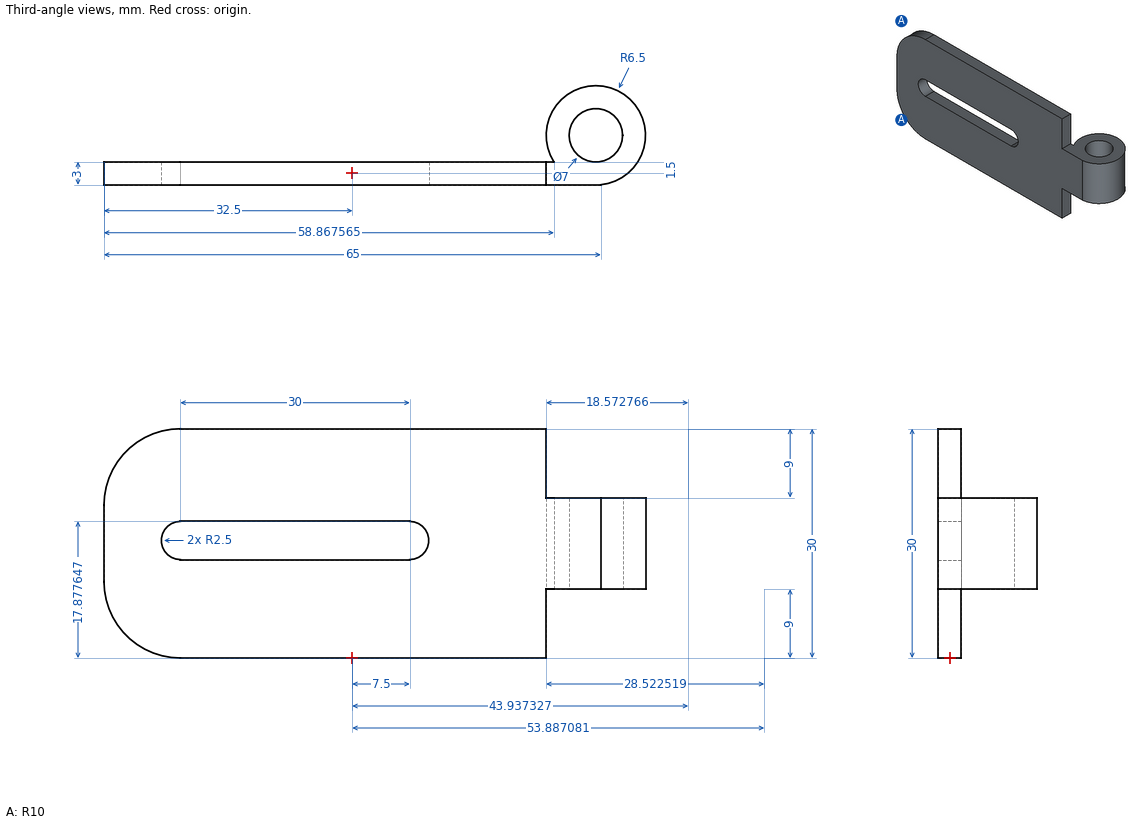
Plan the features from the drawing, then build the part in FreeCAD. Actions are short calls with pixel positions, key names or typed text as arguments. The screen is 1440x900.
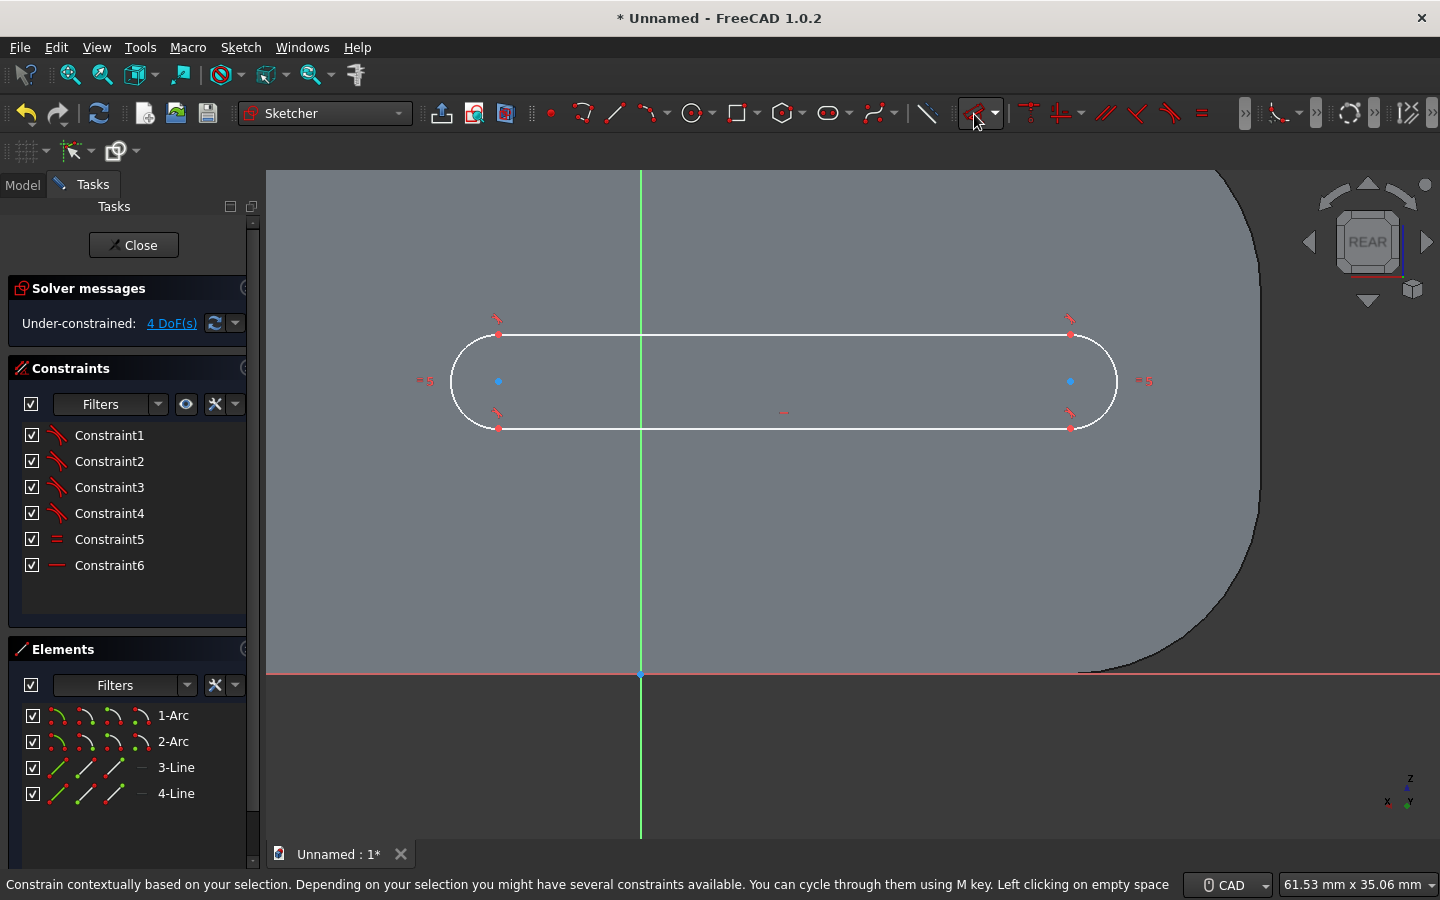
click(460, 354)
click(434, 335)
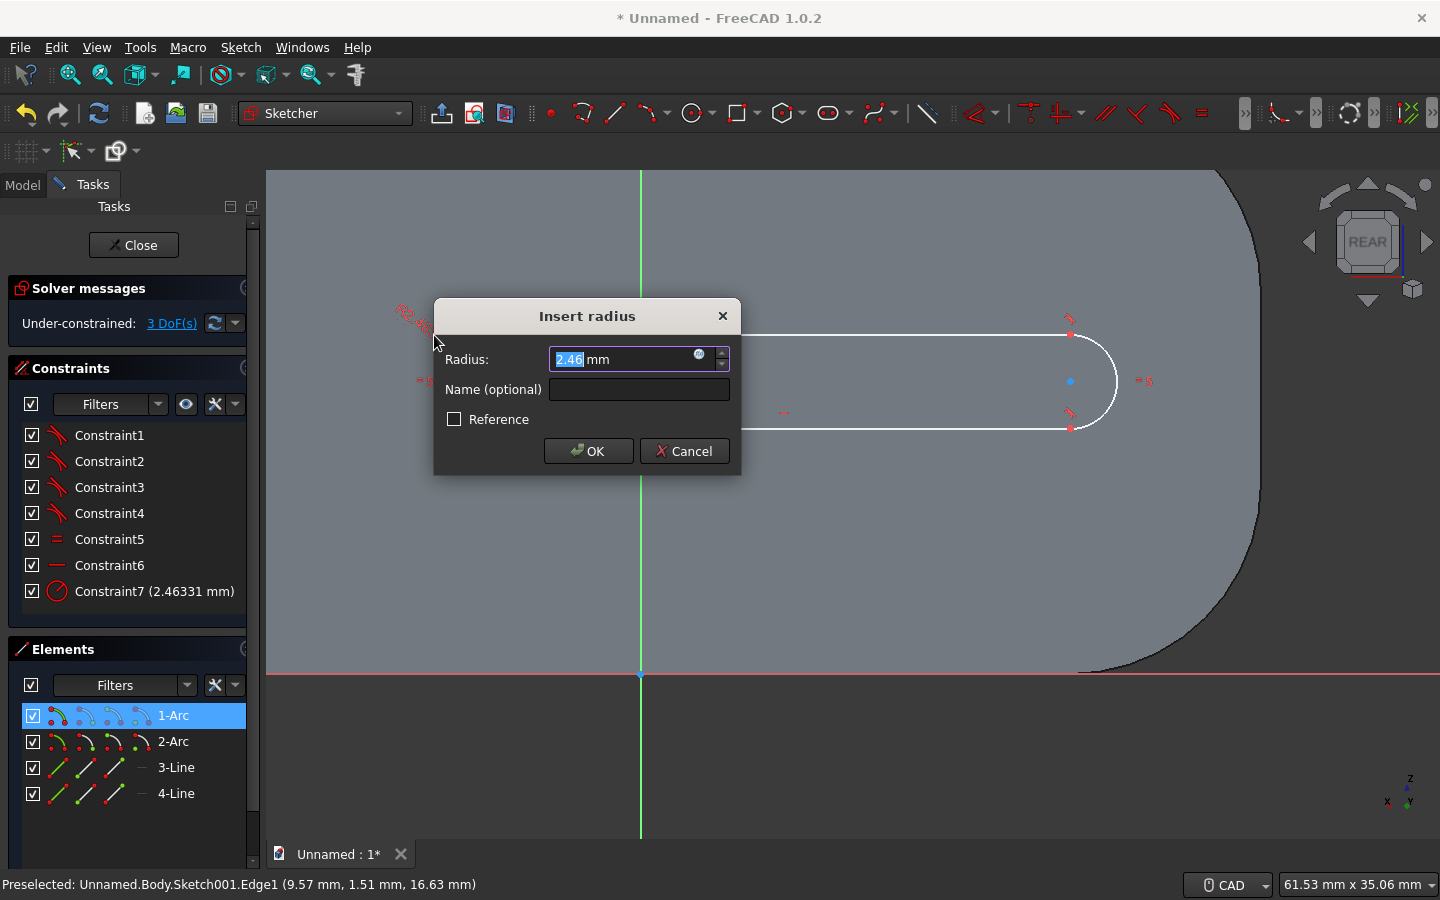
text(2.5)
key(Return)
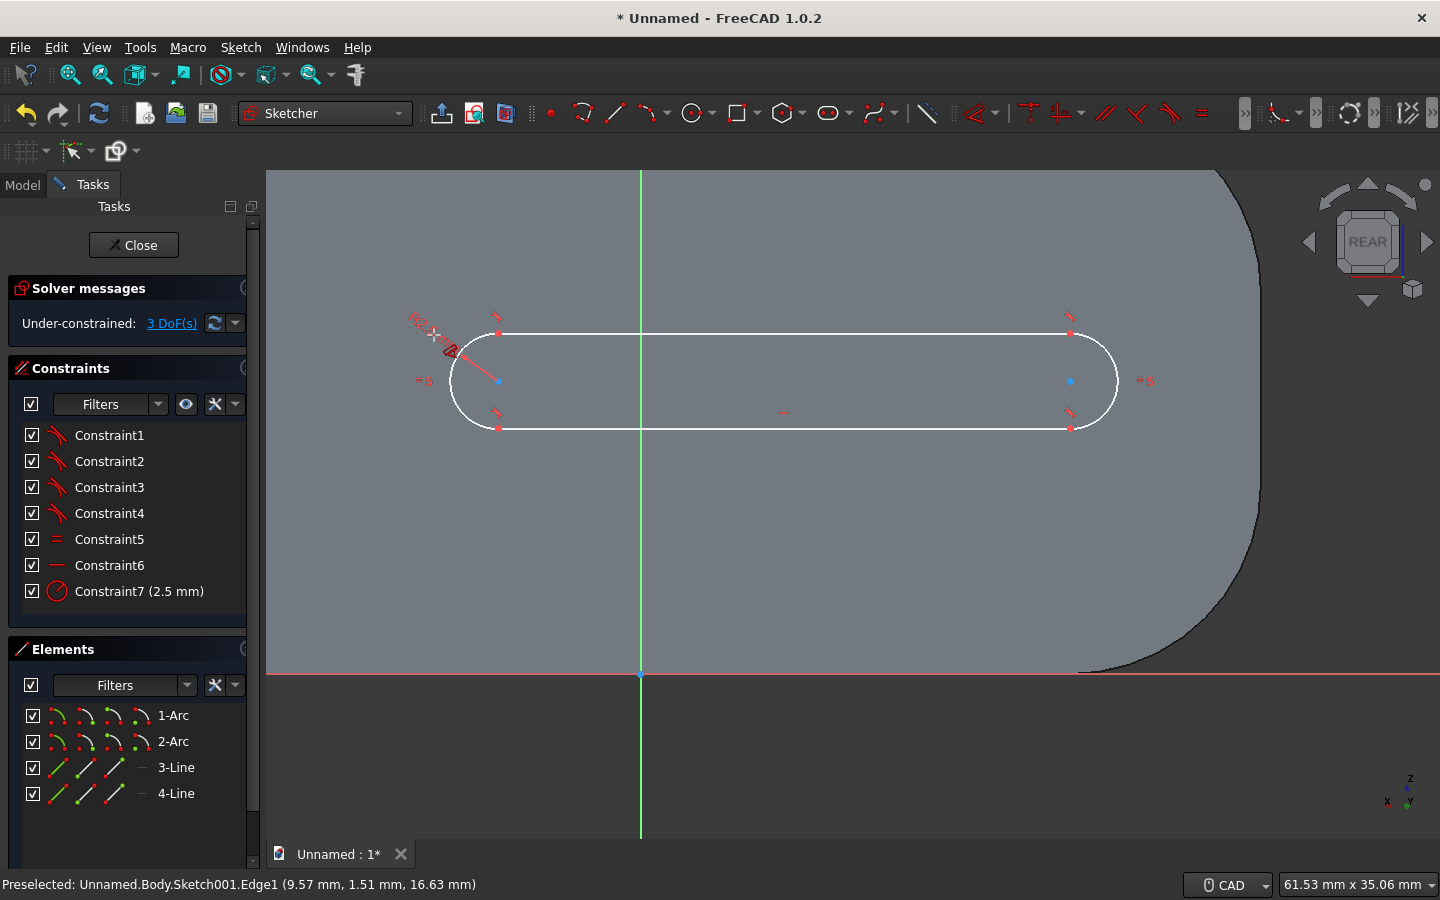
click(670, 334)
click(784, 300)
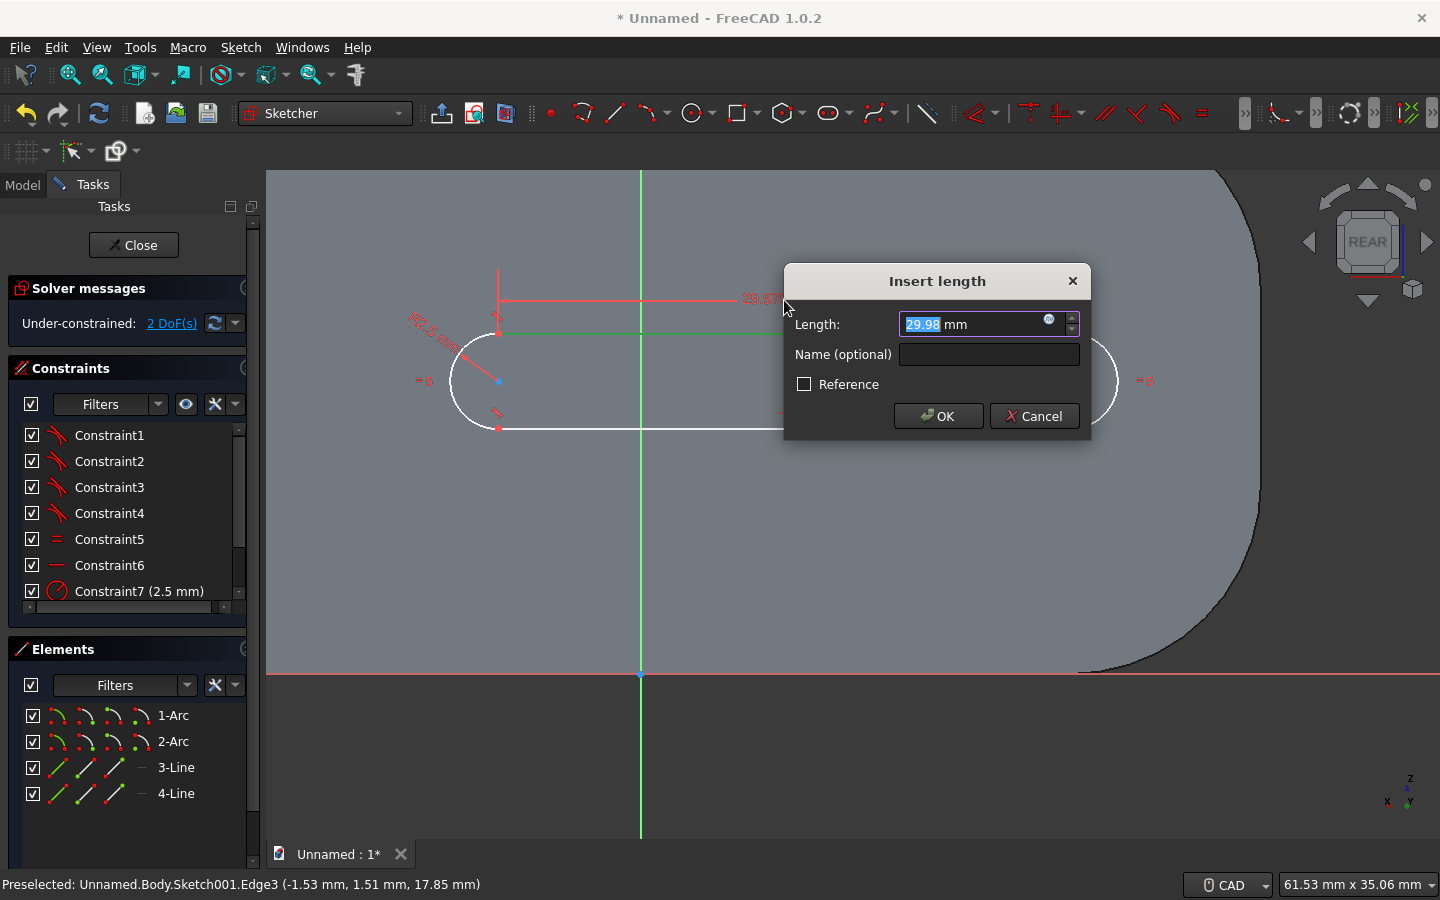
text(30)
key(Return)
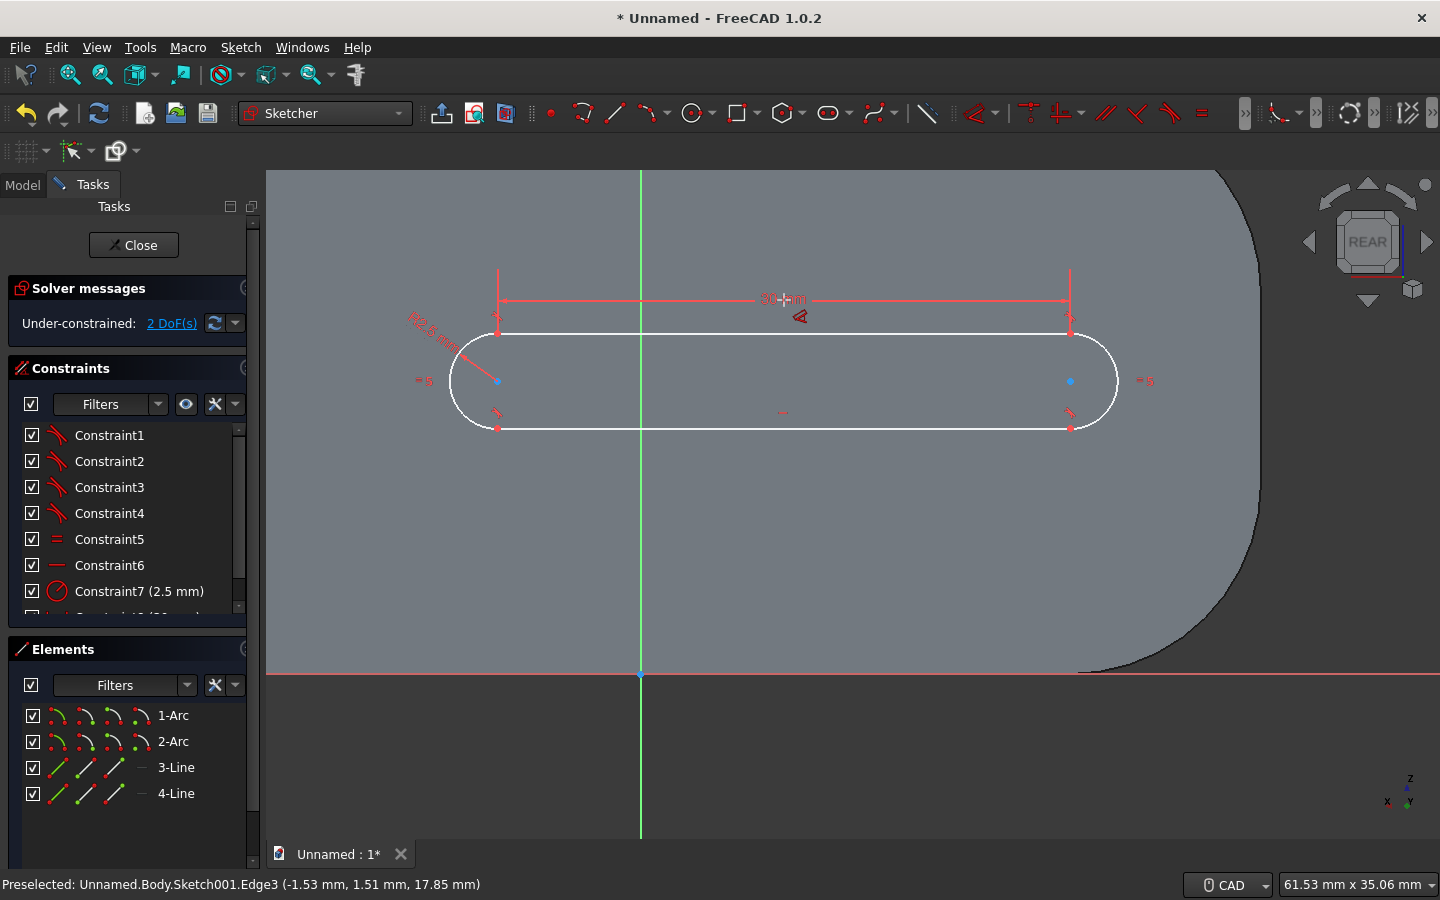
click(498, 334)
click(569, 708)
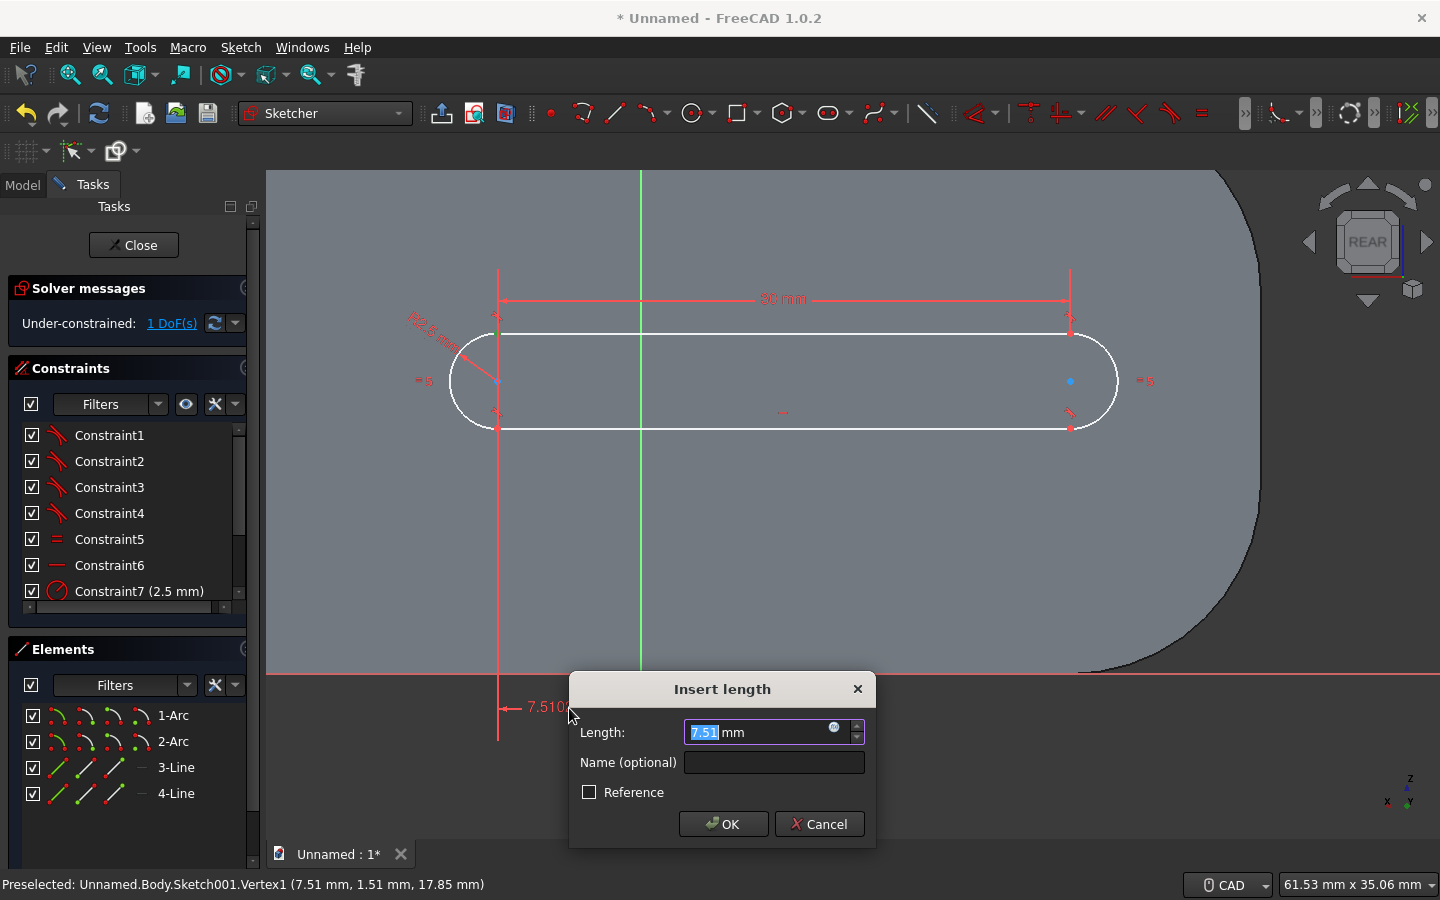
text(7.5)
key(Return)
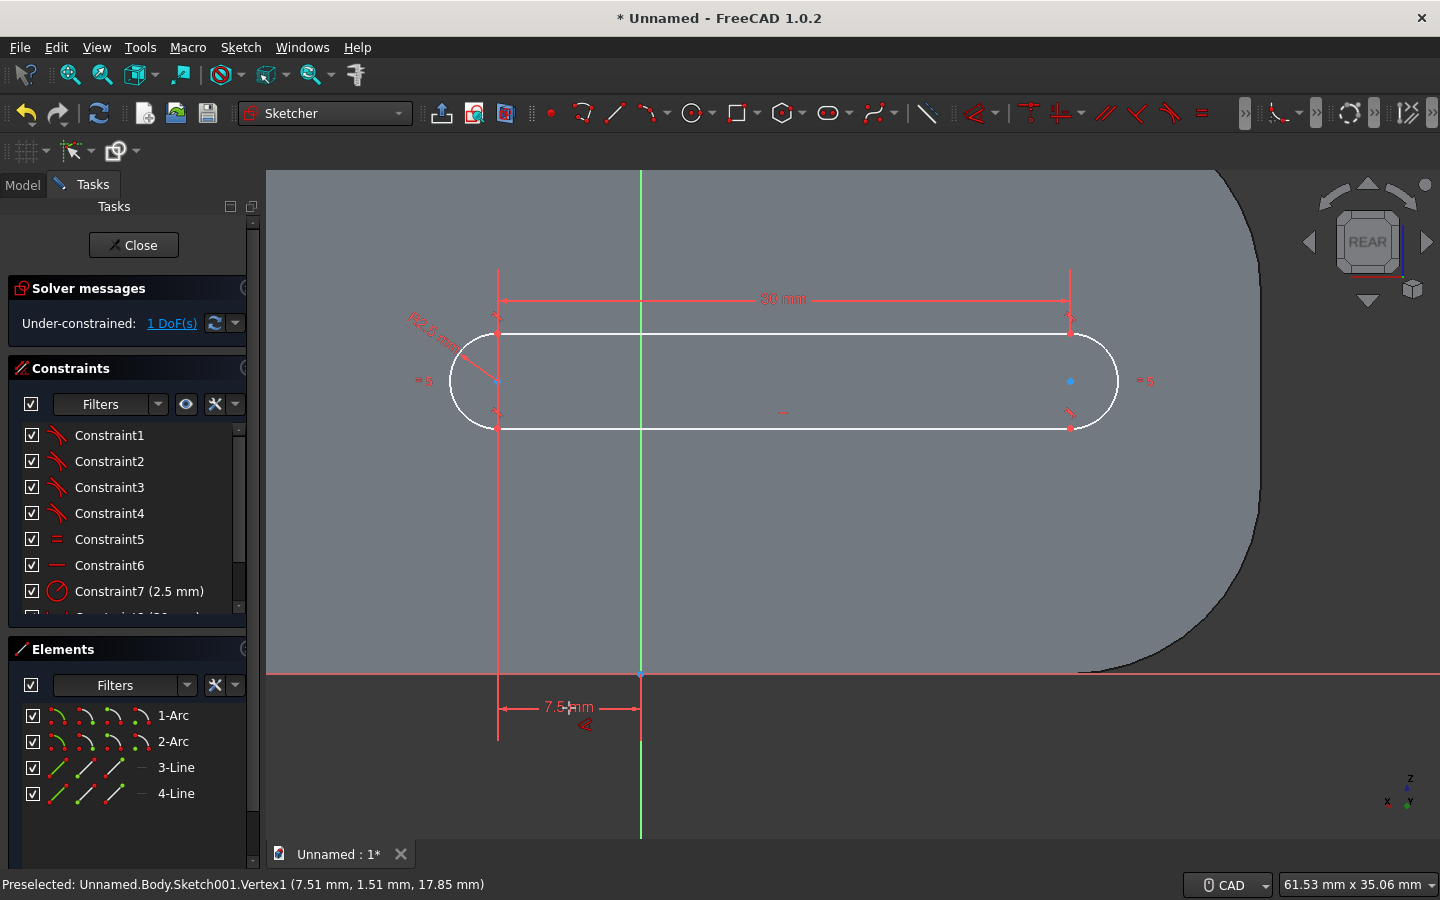
click(498, 334)
click(464, 504)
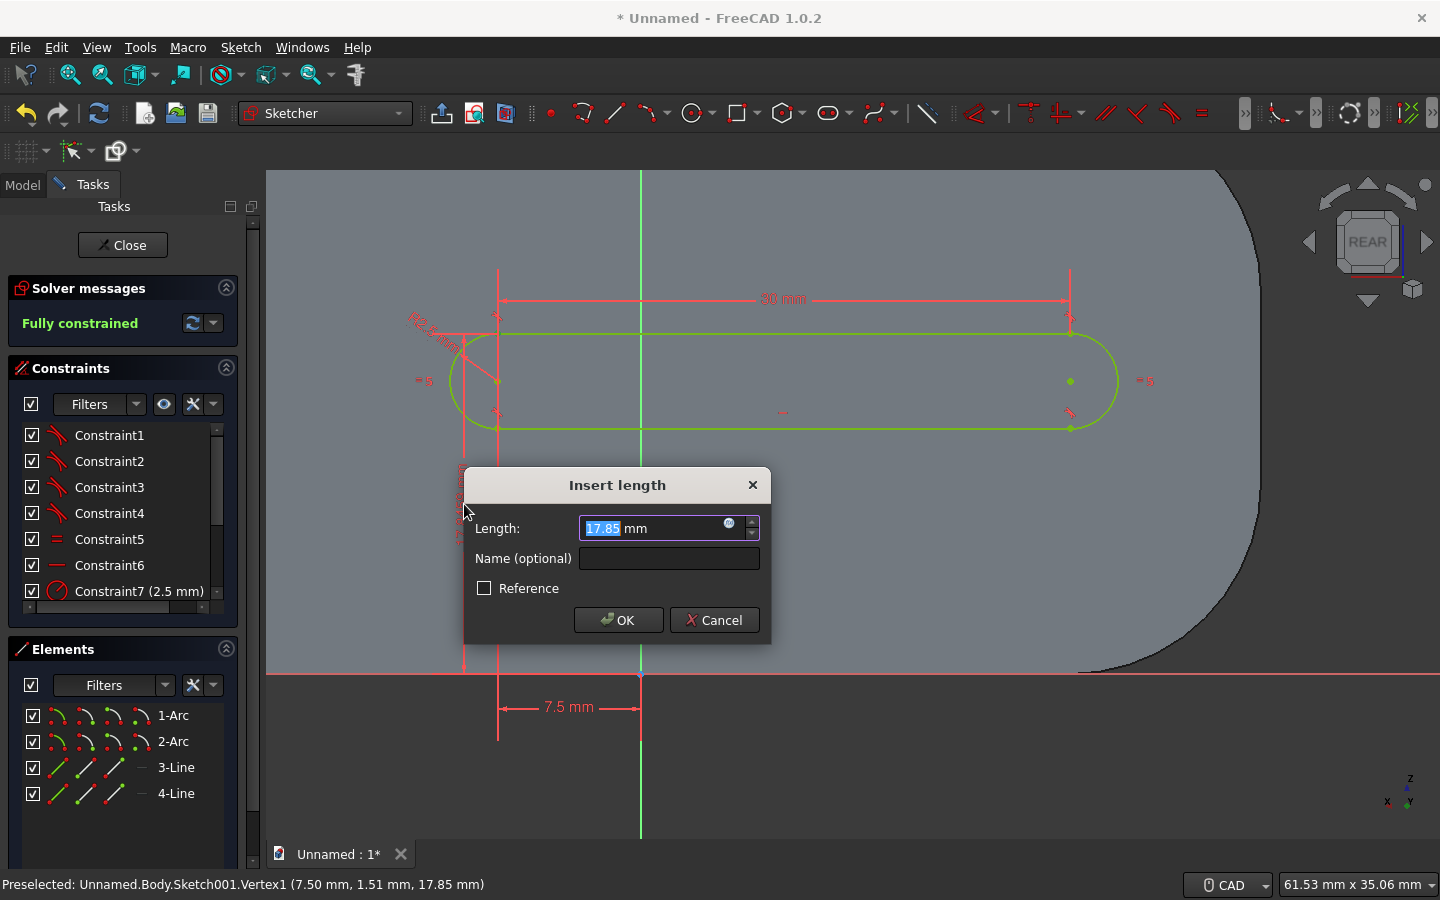
text(17.877647)
key(Return)
key(Escape)